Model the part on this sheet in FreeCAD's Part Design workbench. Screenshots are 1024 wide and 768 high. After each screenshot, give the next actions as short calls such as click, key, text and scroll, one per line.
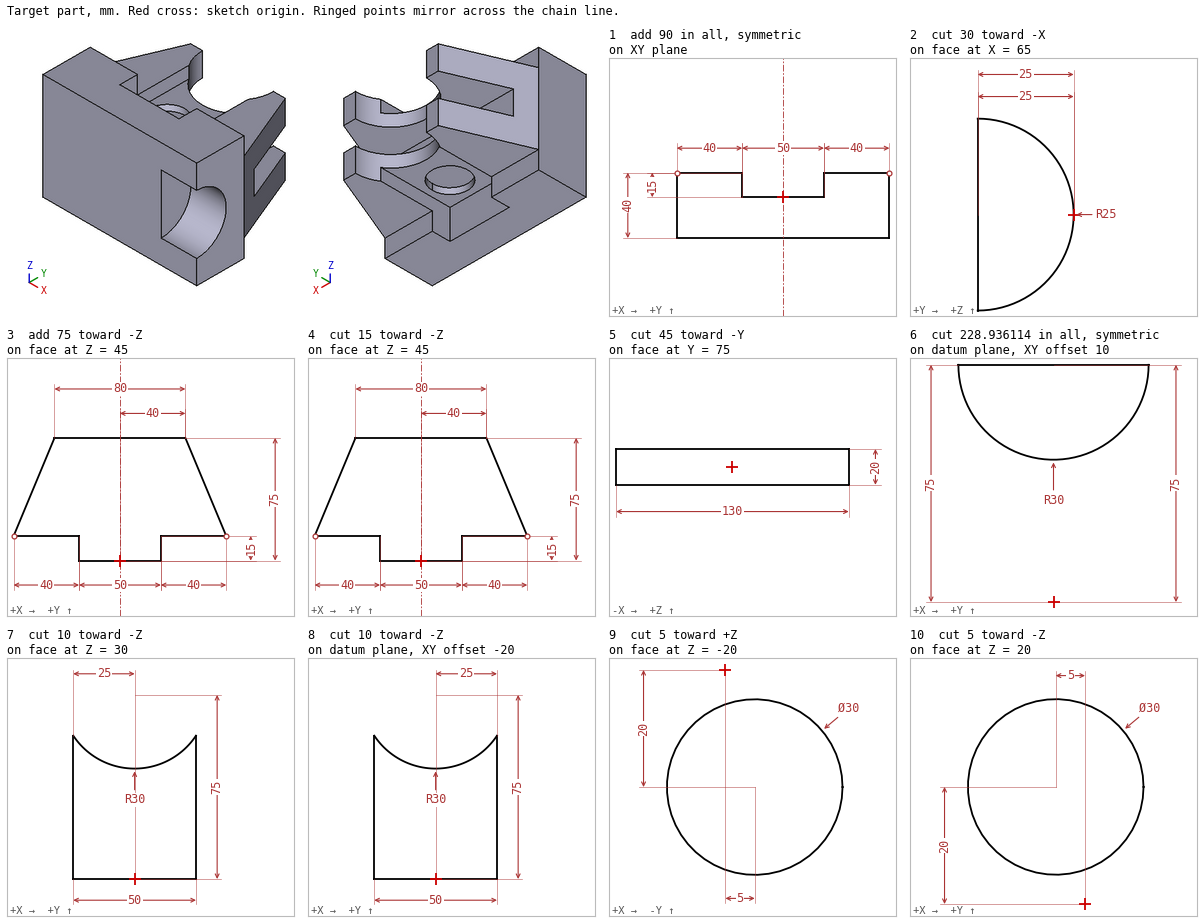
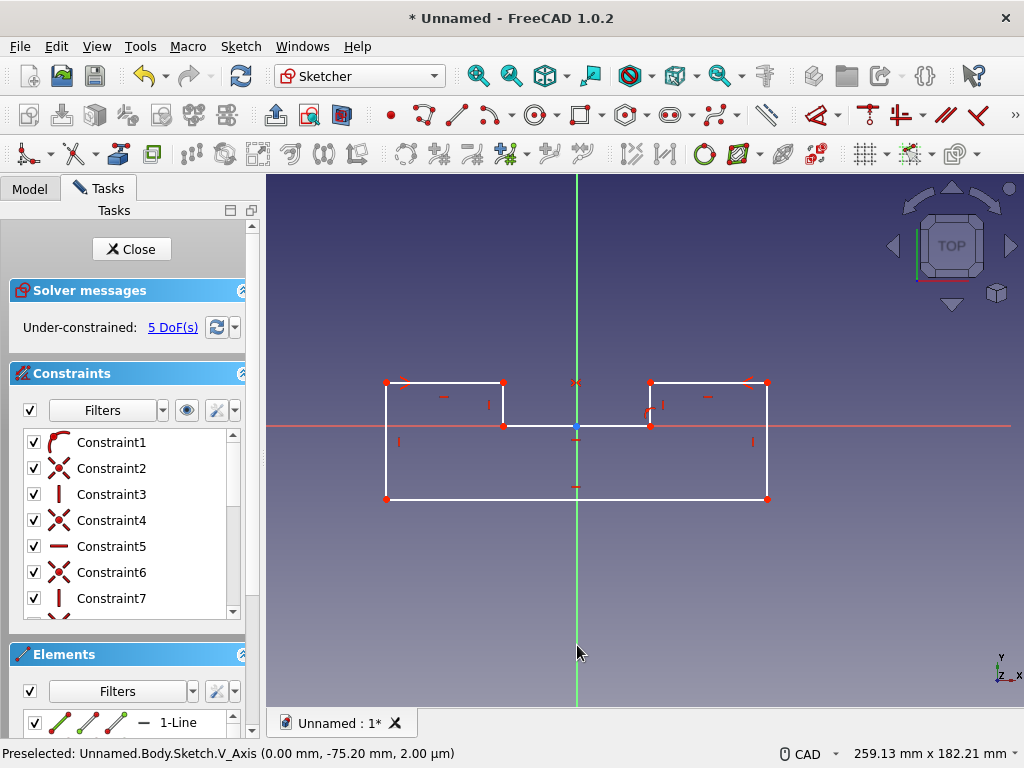
key(d)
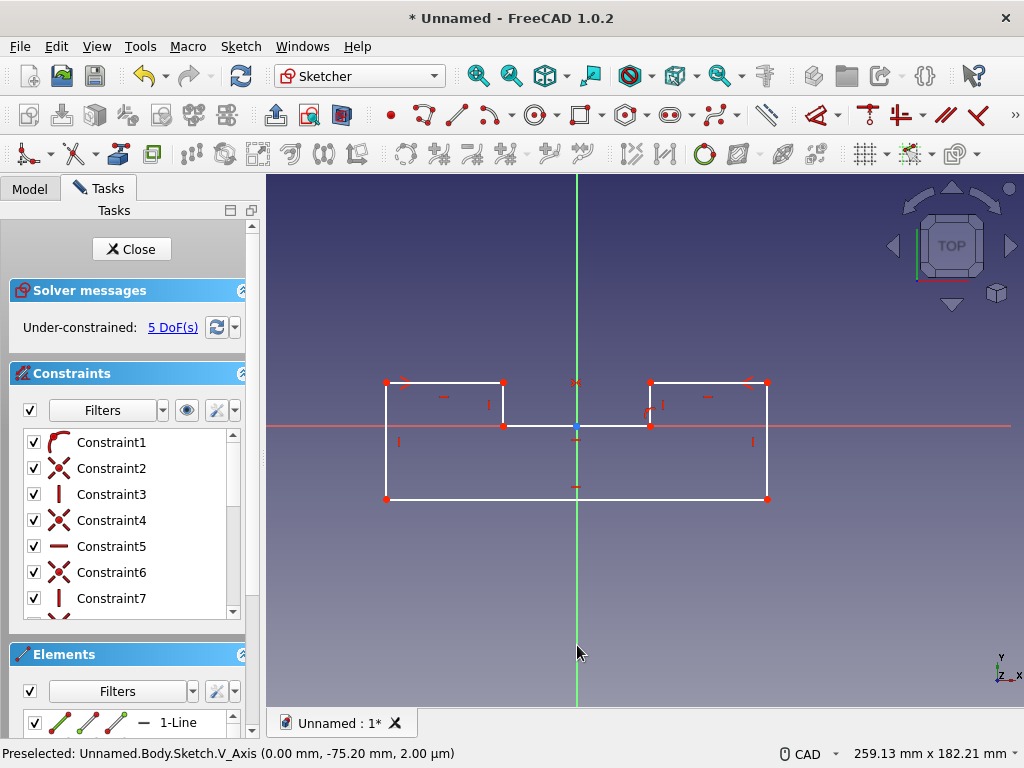
click(606, 426)
click(543, 392)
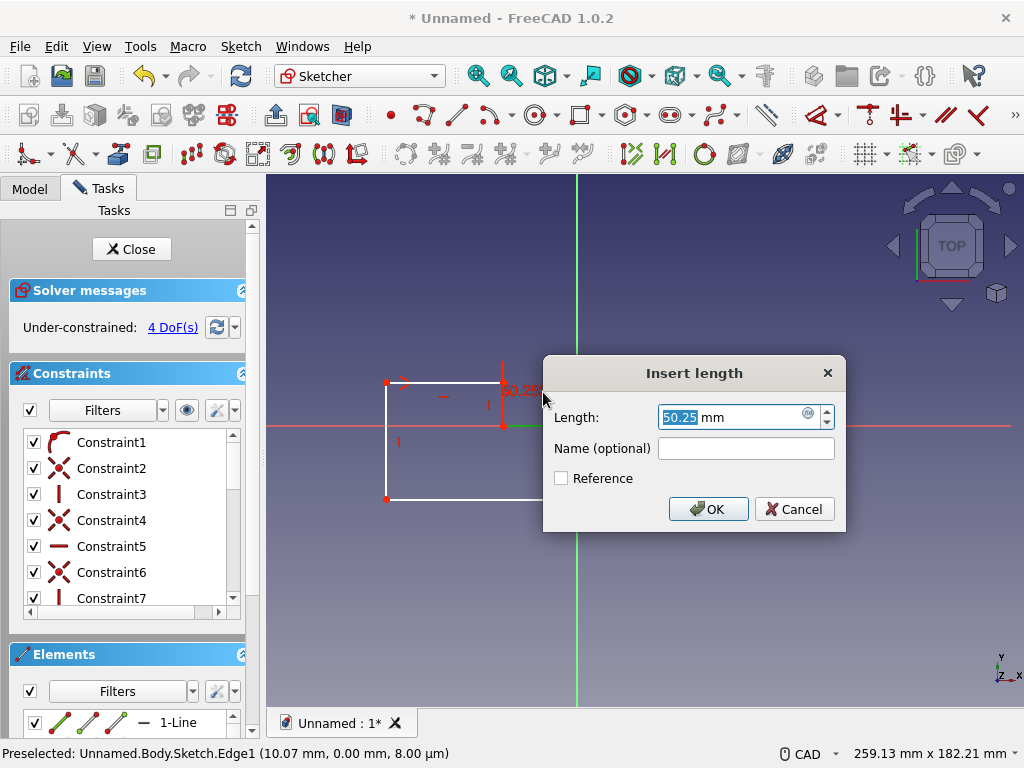
text(50)
key(Return)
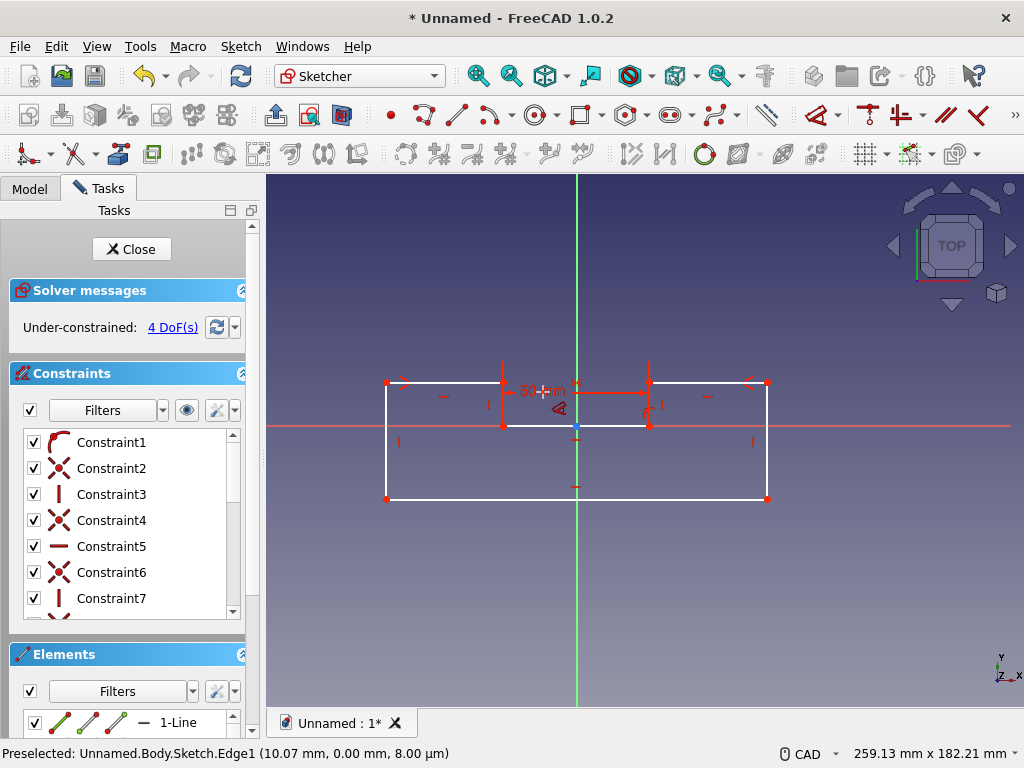
click(503, 413)
click(469, 405)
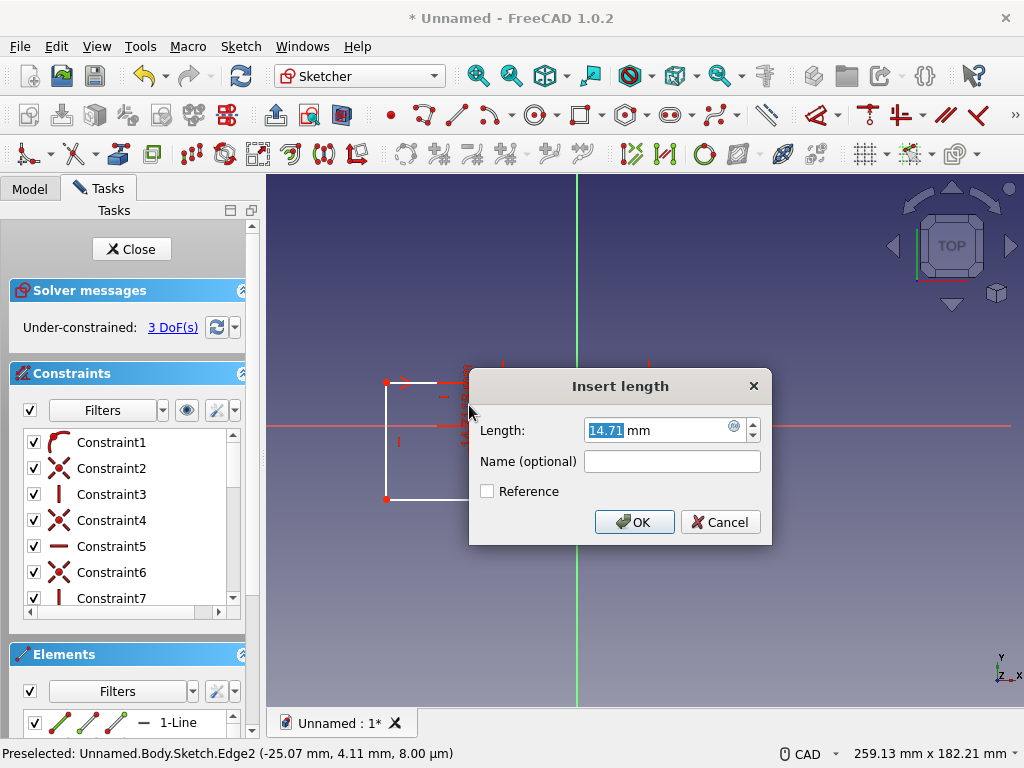
text(15)
key(Return)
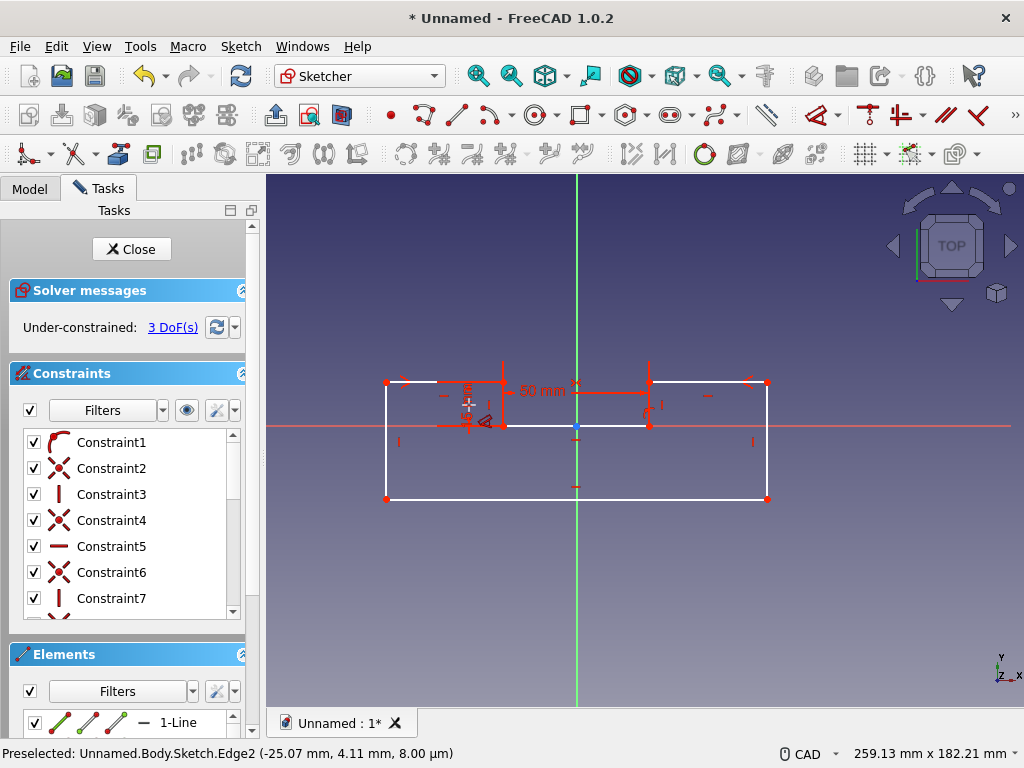
click(468, 382)
click(445, 348)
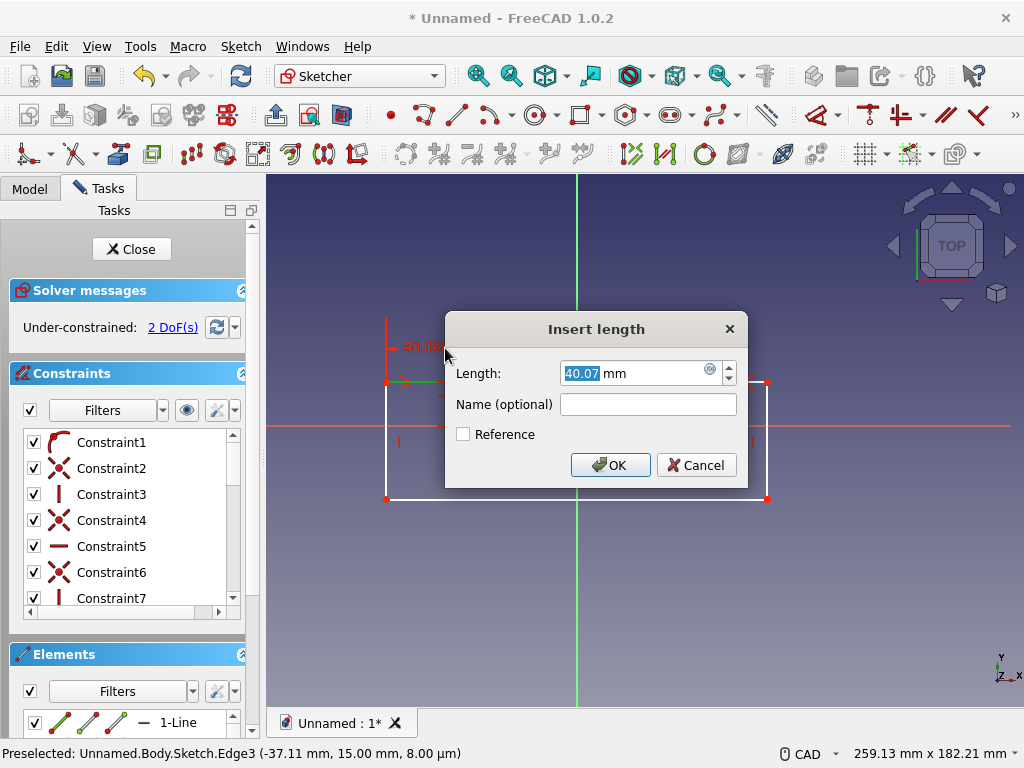
text(40)
key(Return)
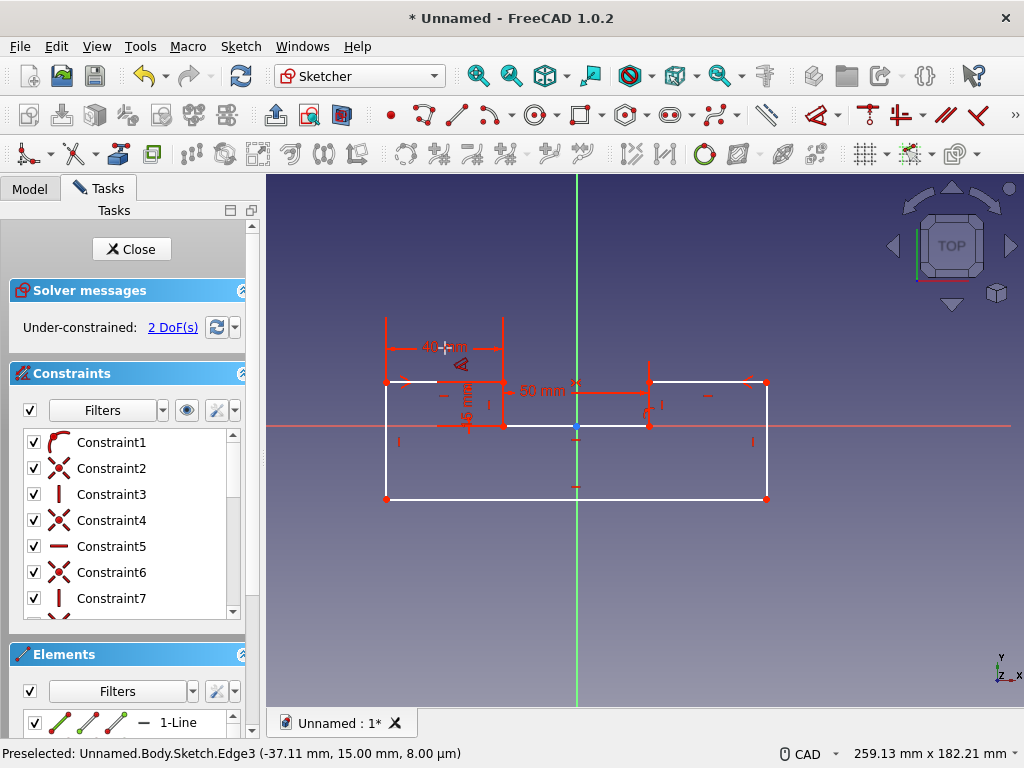
click(386, 465)
click(352, 441)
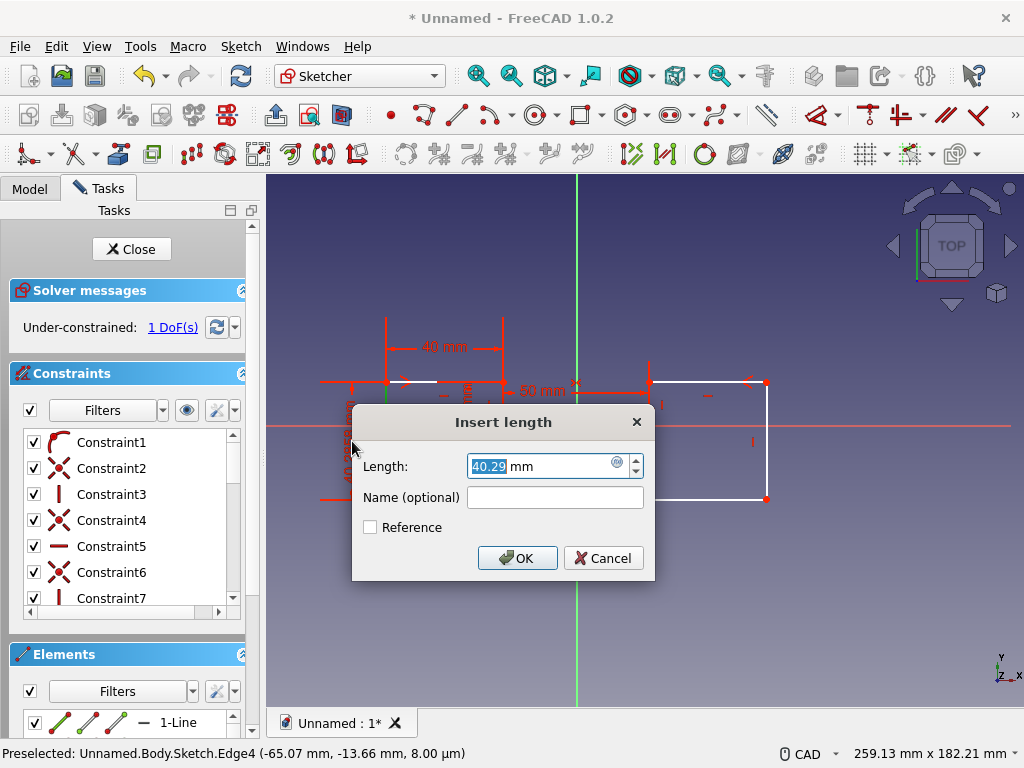
text(40)
key(Return)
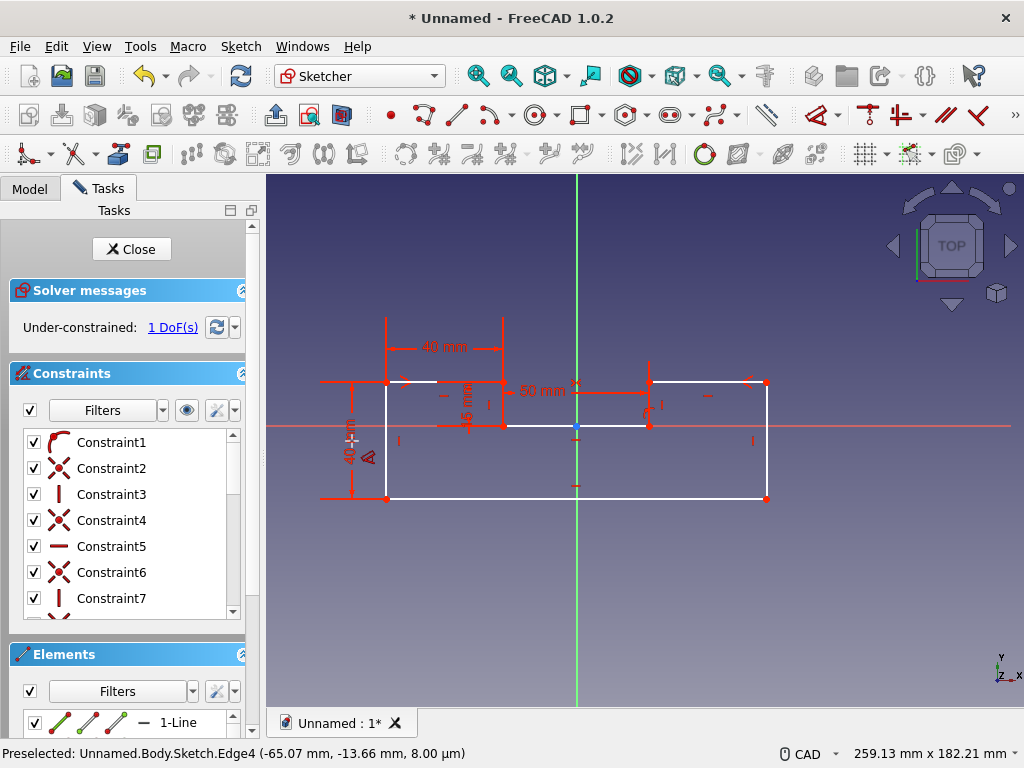
click(732, 382)
click(708, 348)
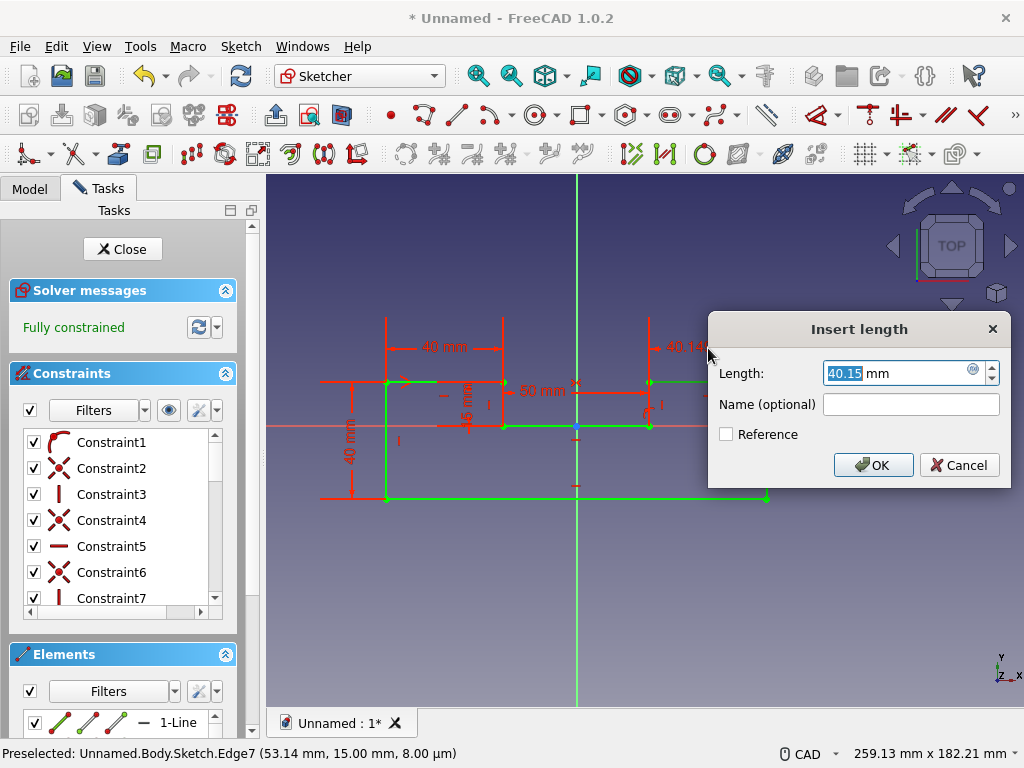
text(40)
key(Return)
key(Escape)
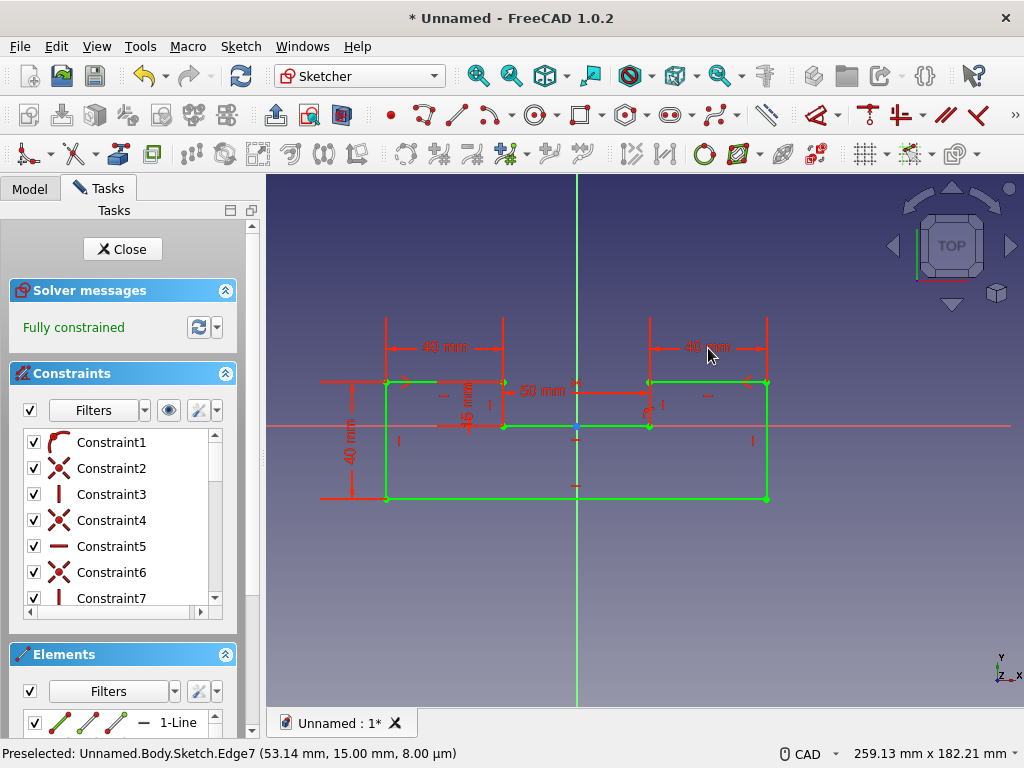
click(123, 249)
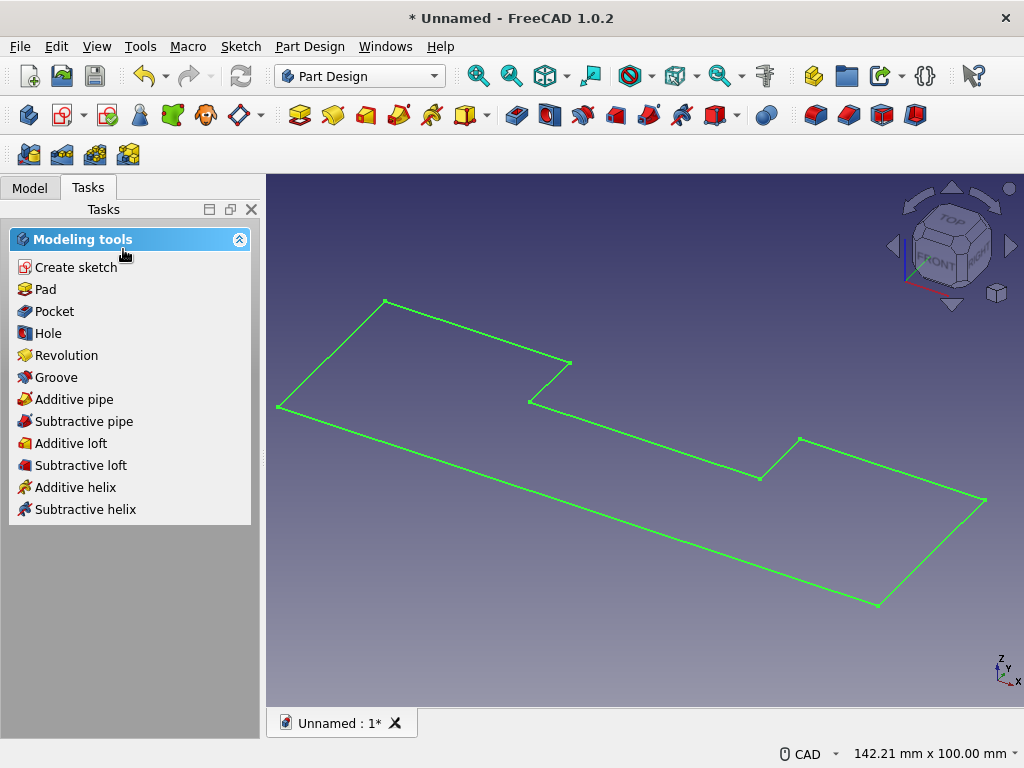
click(300, 116)